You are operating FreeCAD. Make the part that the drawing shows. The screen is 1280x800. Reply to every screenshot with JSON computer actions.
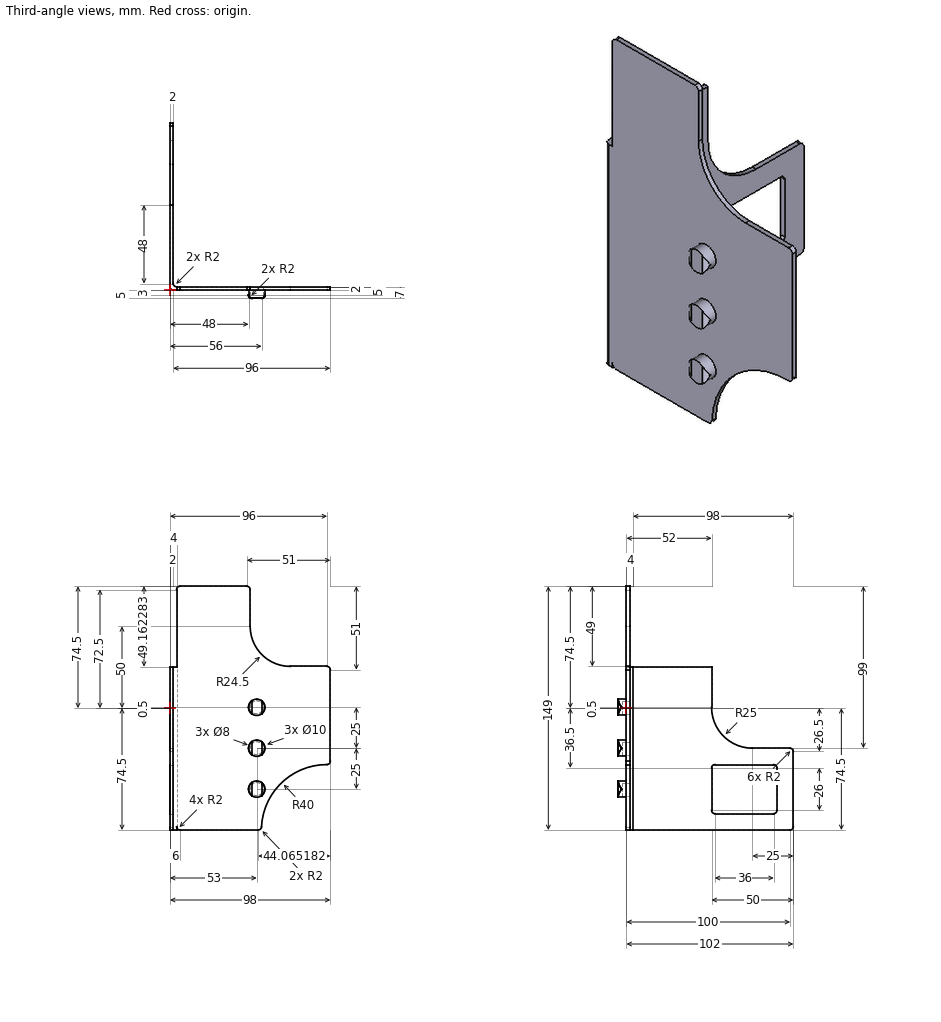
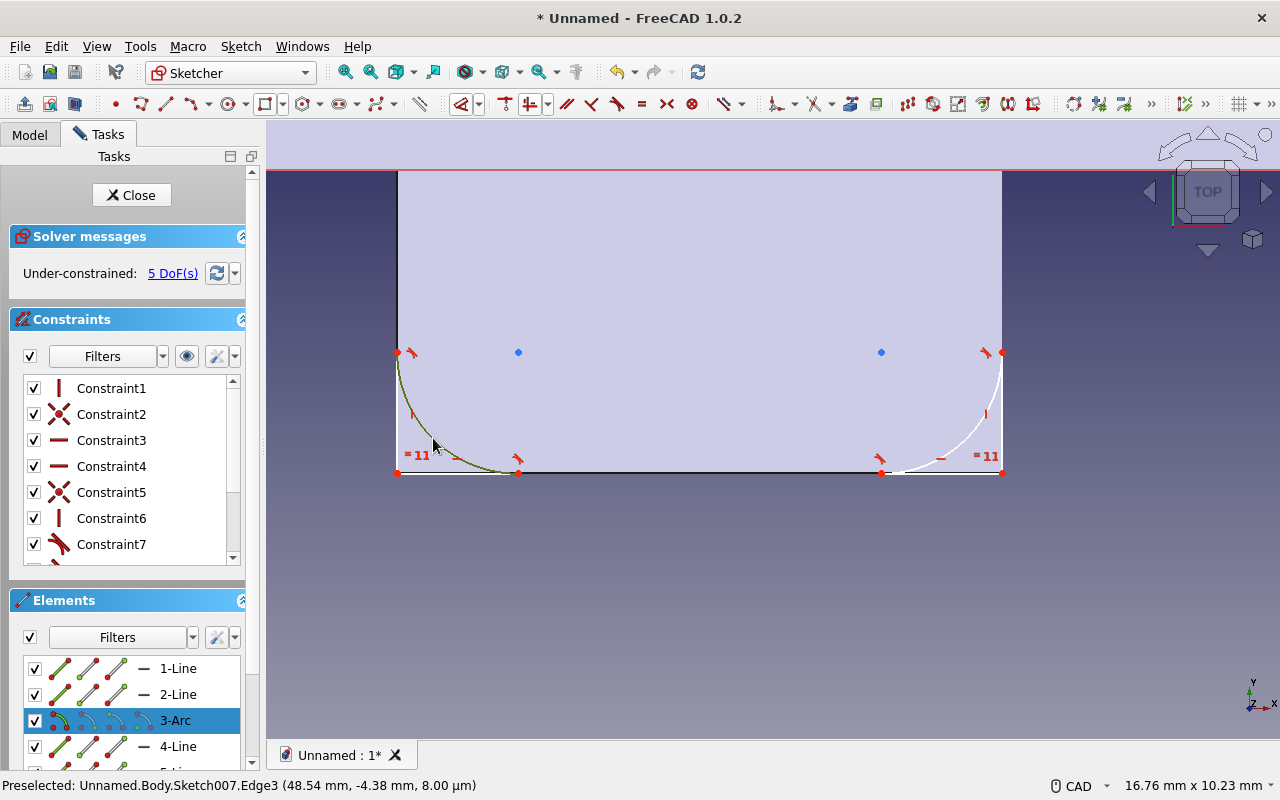
{"action": "key", "text": "k r"}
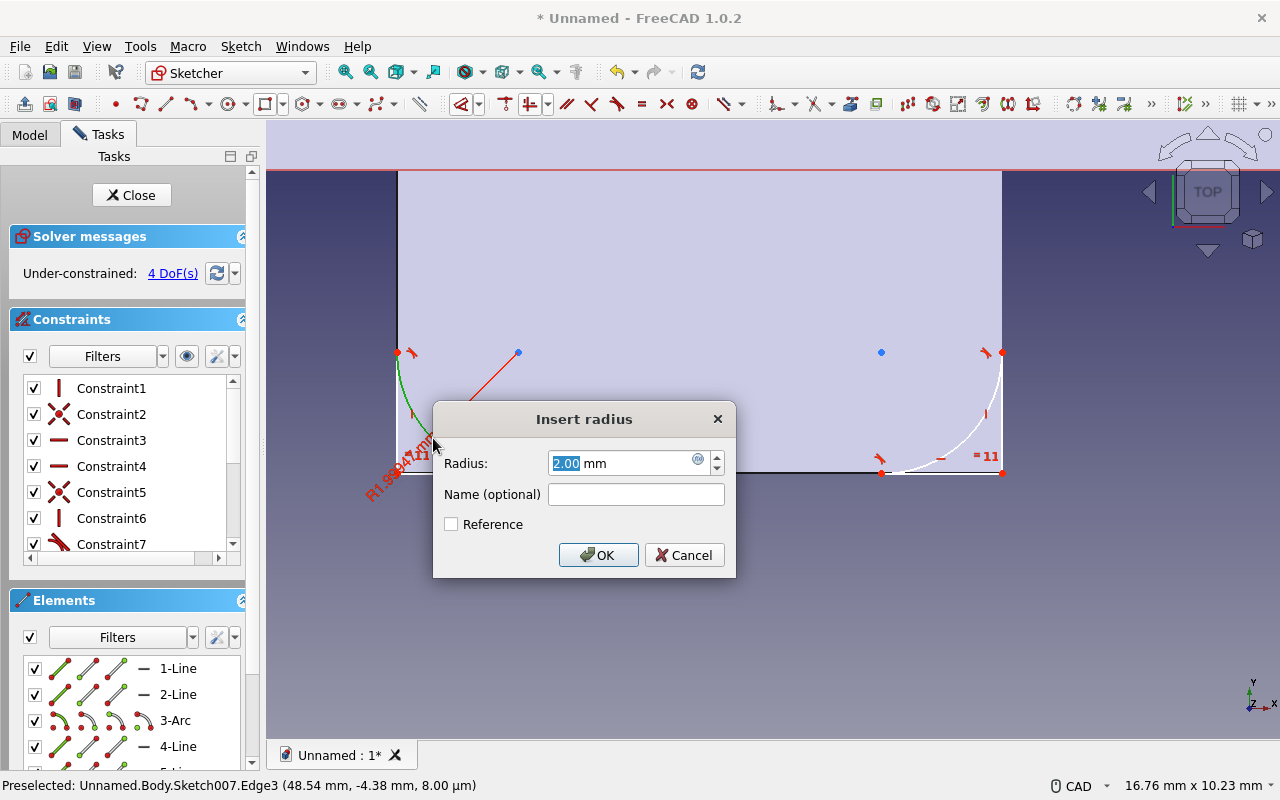
{"action": "type", "text": "2"}
{"action": "key", "text": "Return"}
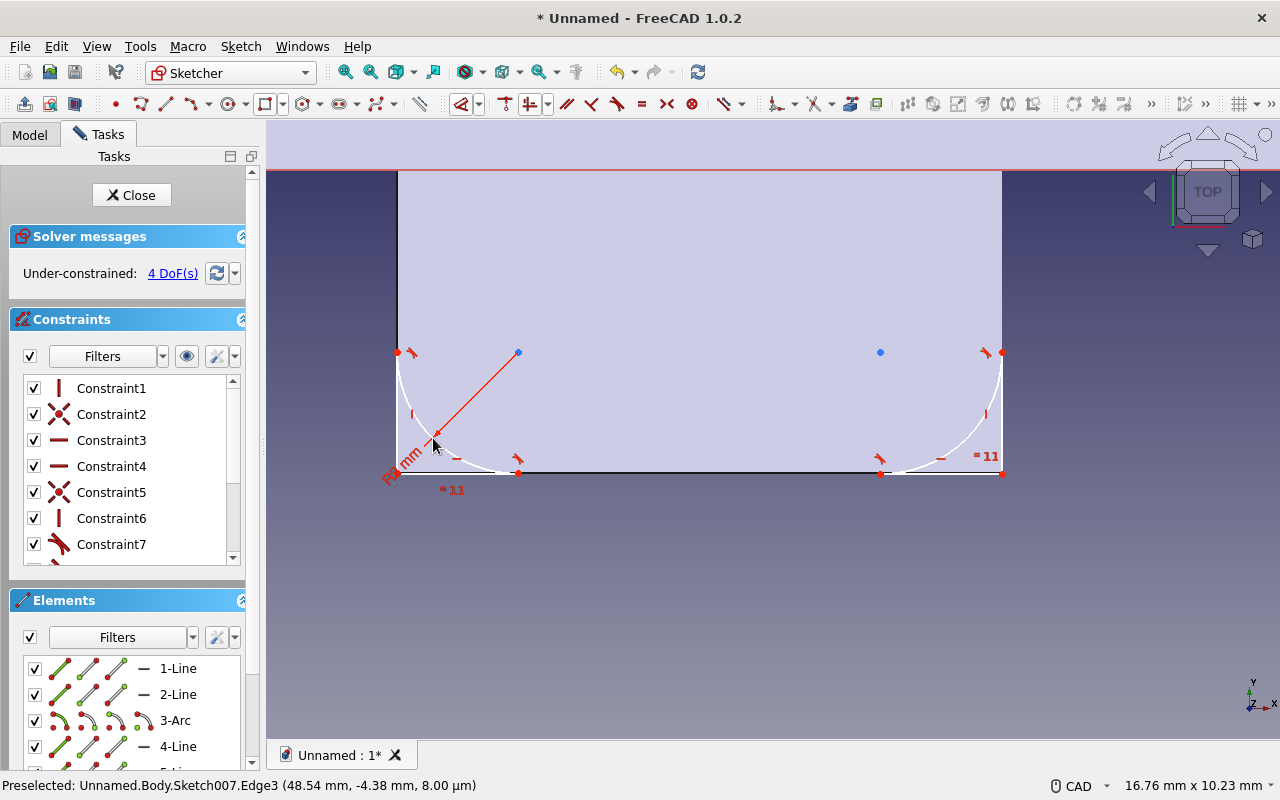
{"action": "left_click", "coordinate": [397, 353]}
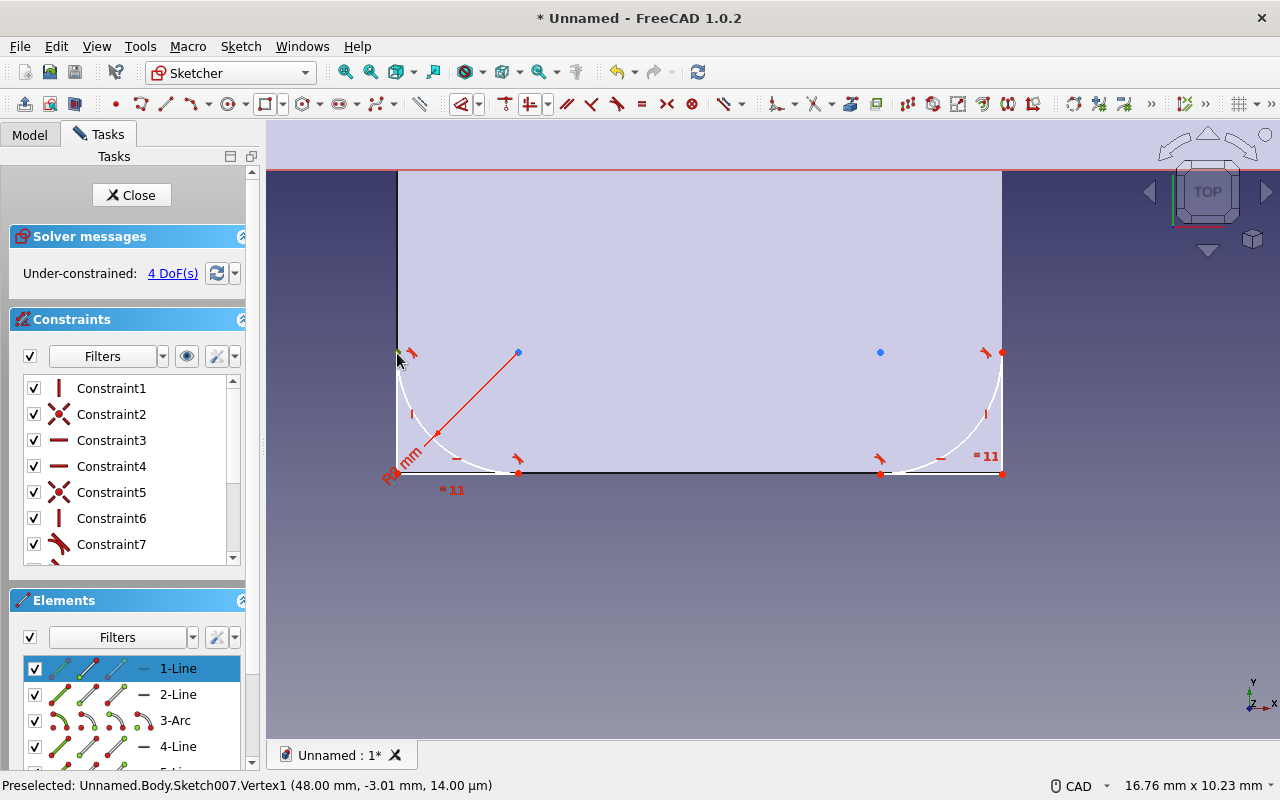
{"action": "key", "text": "i"}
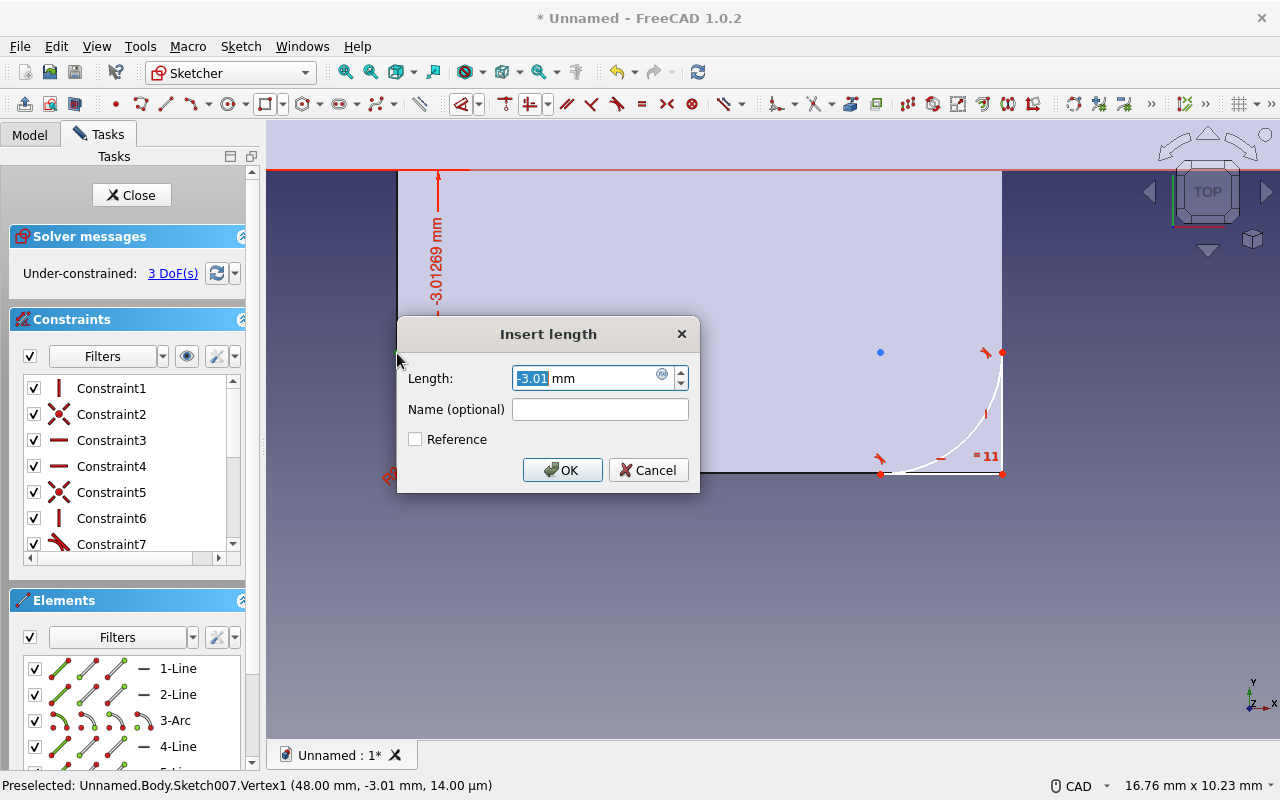
{"action": "type", "text": "-3"}
{"action": "key", "text": "Return"}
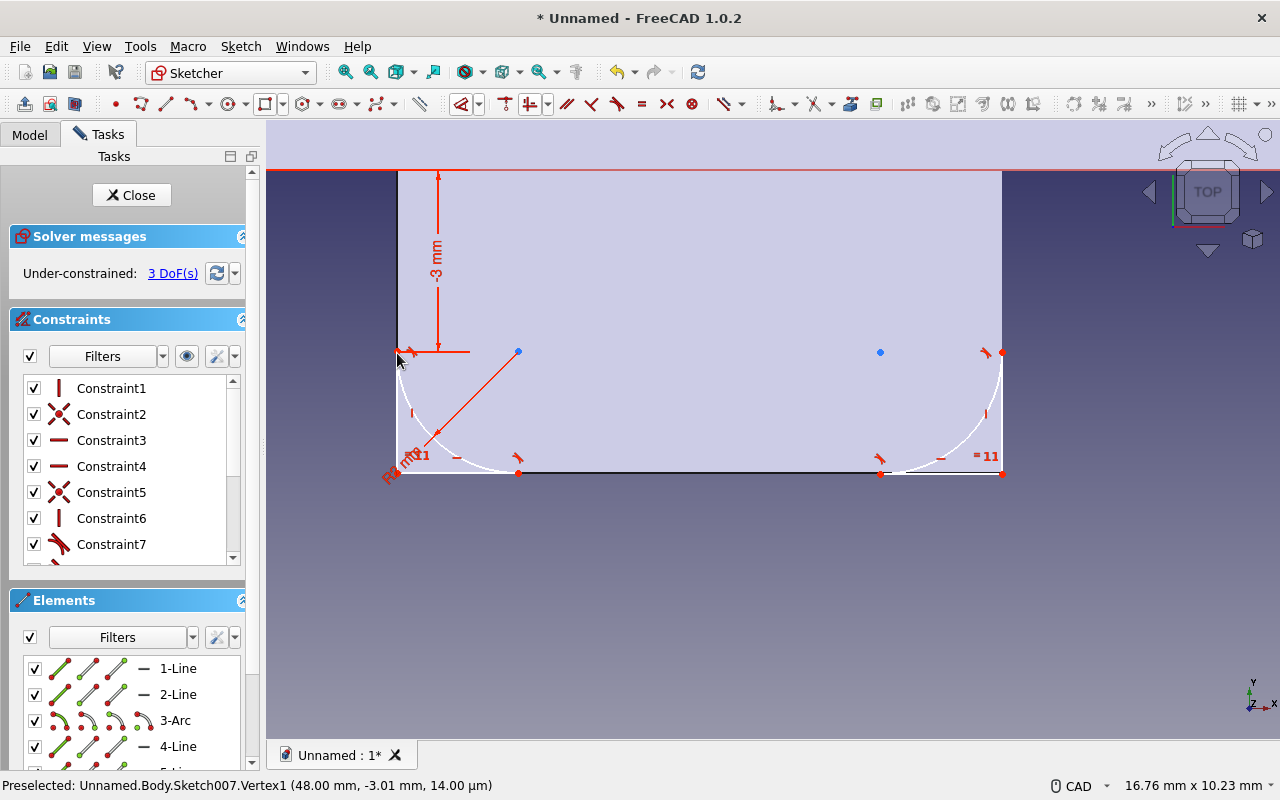
{"action": "left_click", "coordinate": [881, 474]}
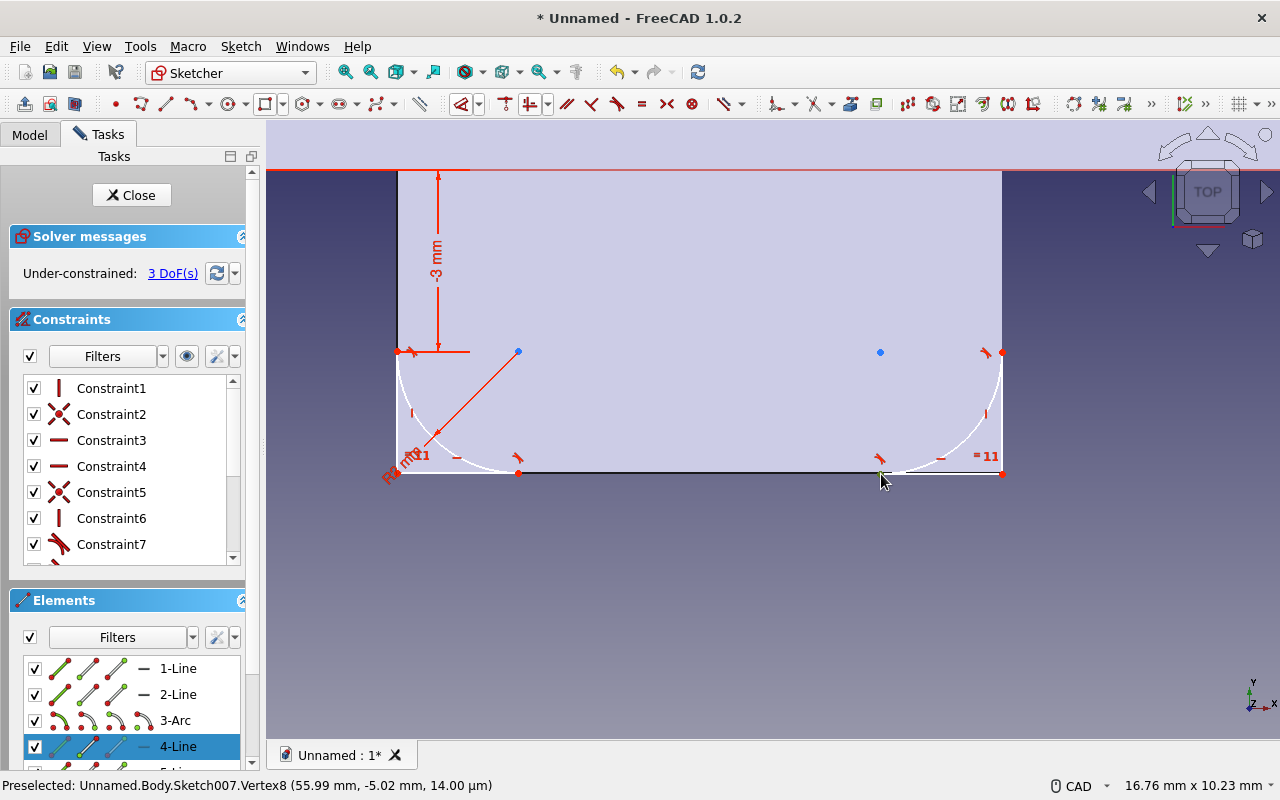
{"action": "key", "text": "i"}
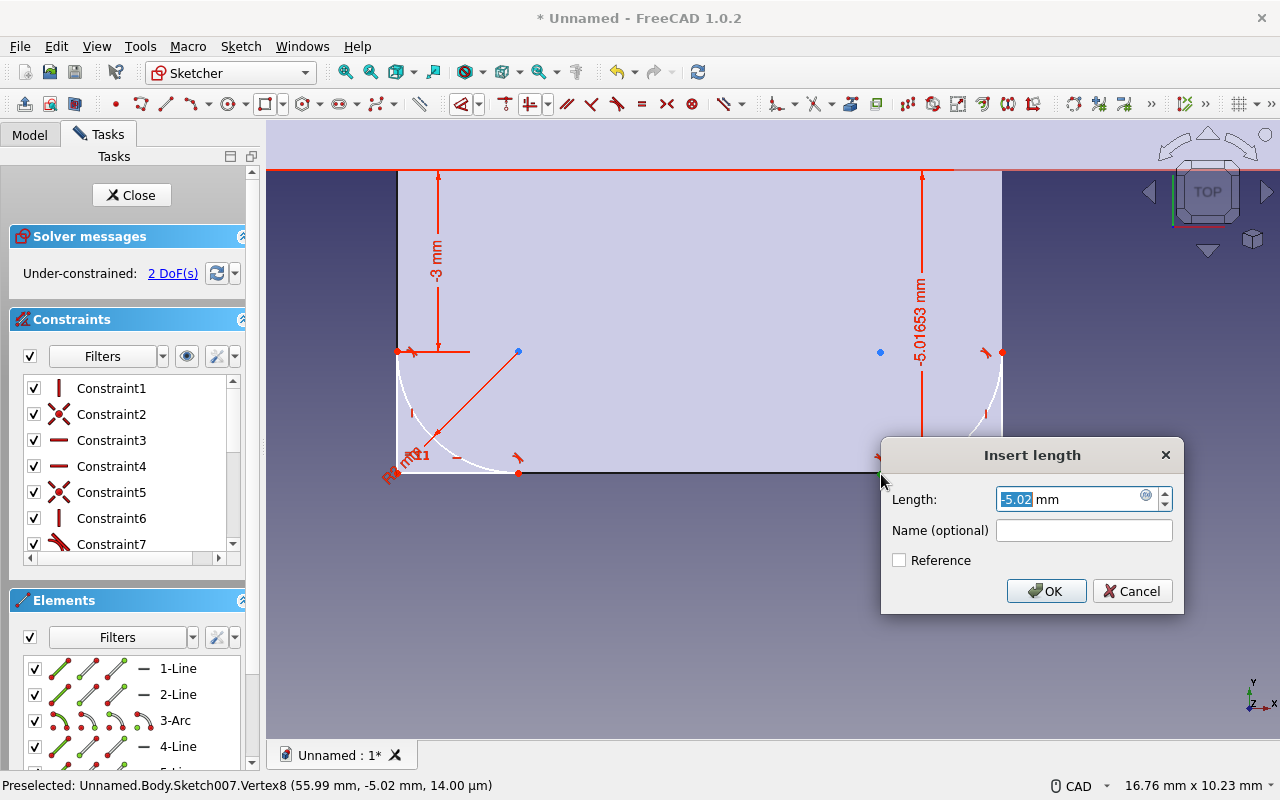
{"action": "type", "text": "-5"}
{"action": "key", "text": "Return"}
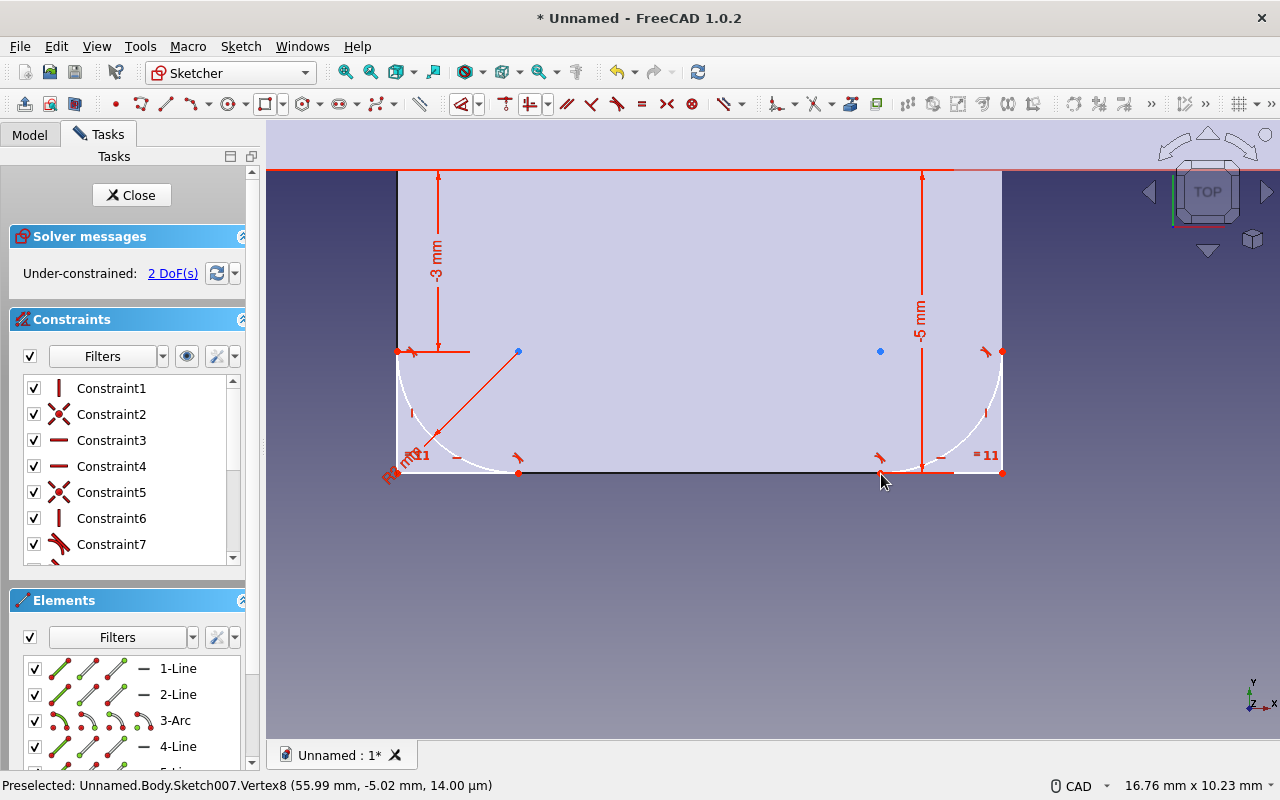
{"action": "left_click", "coordinate": [397, 352]}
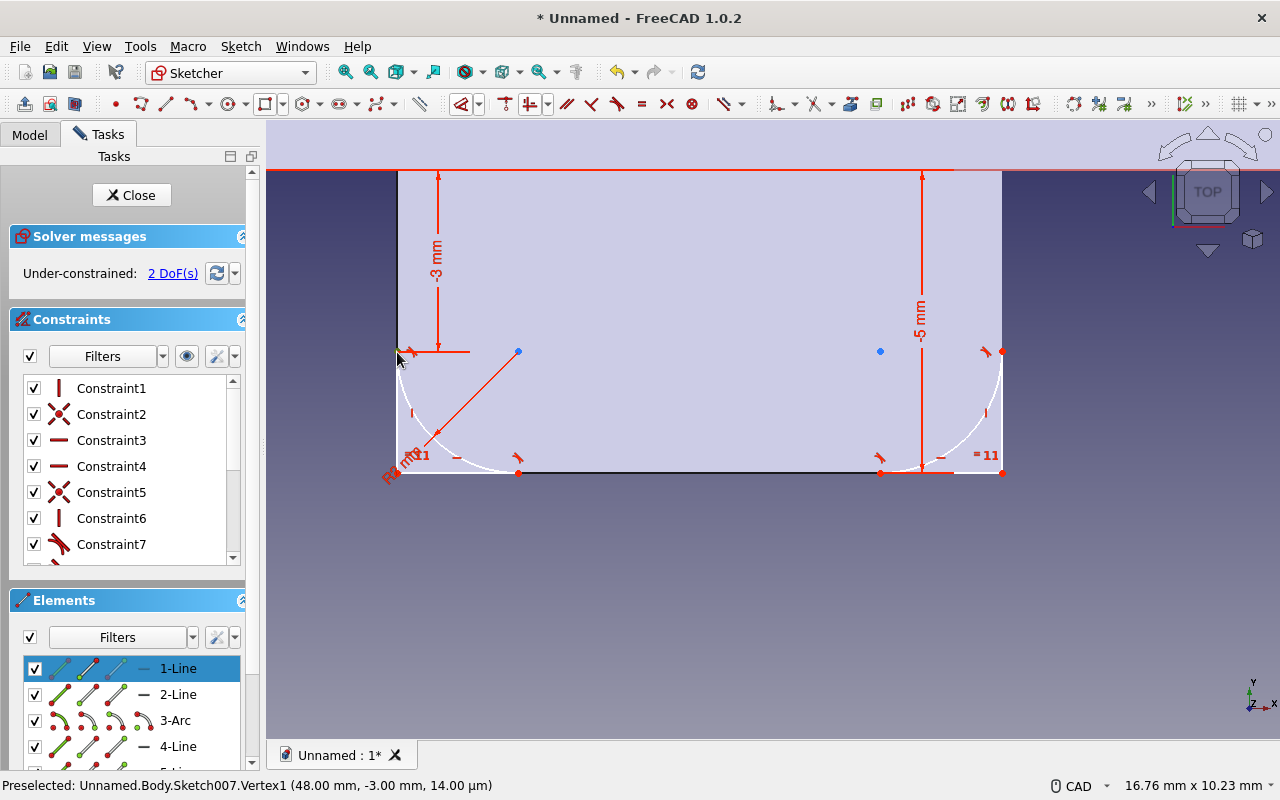
{"action": "key", "text": "l"}